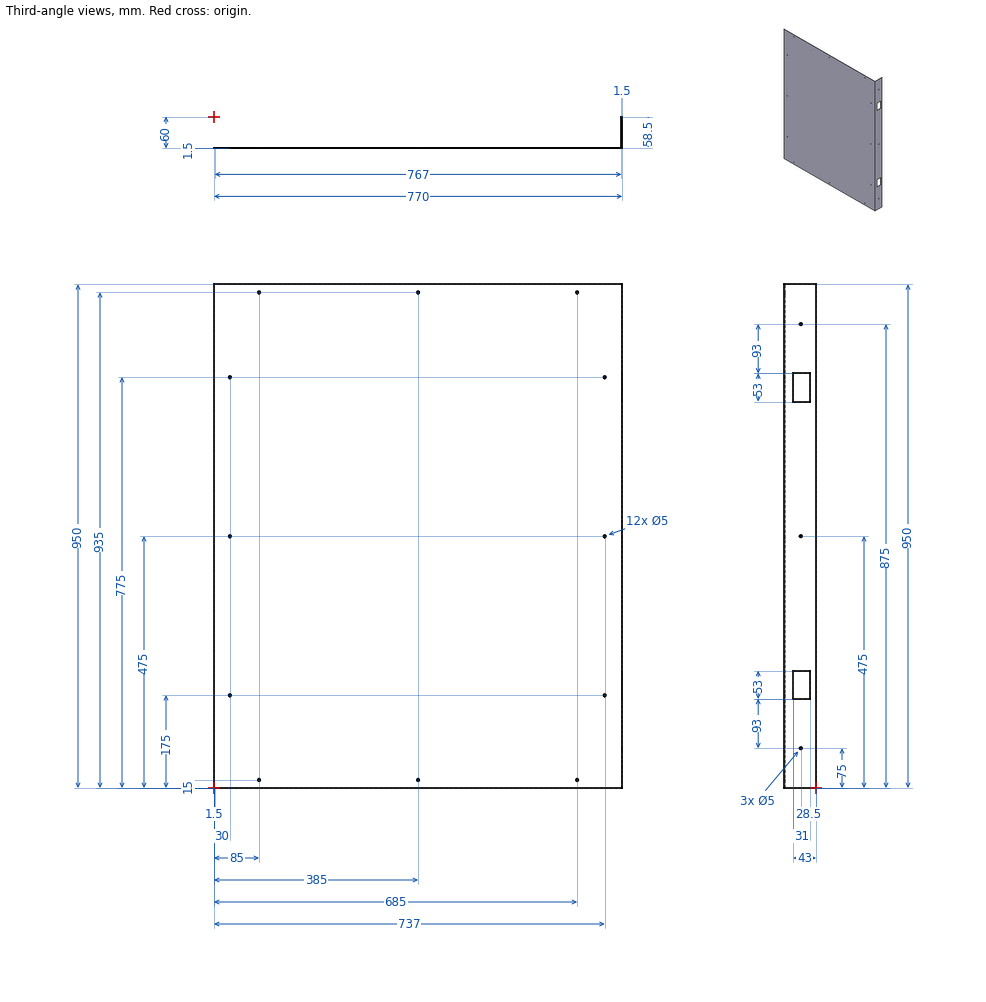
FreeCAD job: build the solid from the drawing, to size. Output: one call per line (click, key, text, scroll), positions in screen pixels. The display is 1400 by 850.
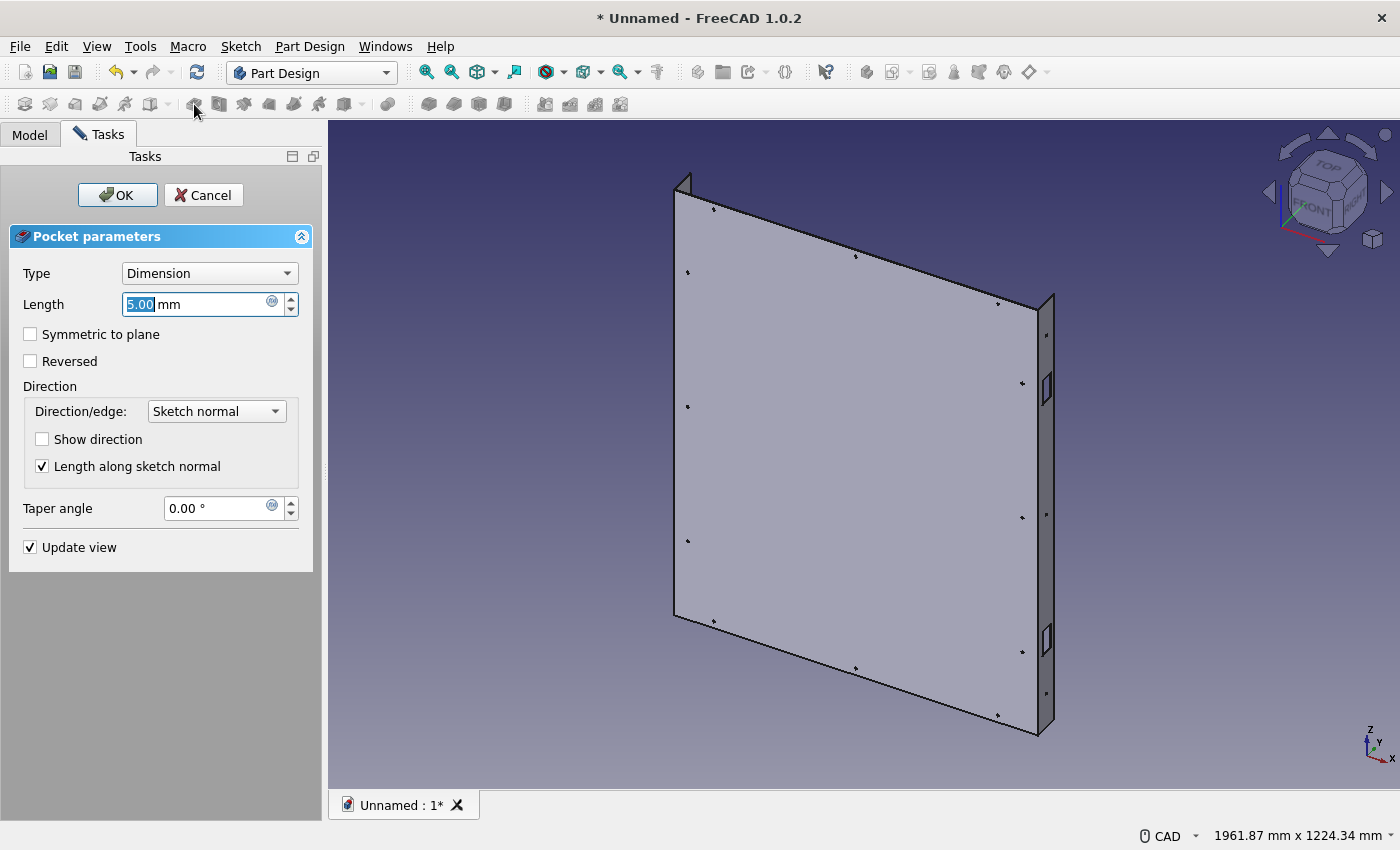
text(58.5)
key(Tab)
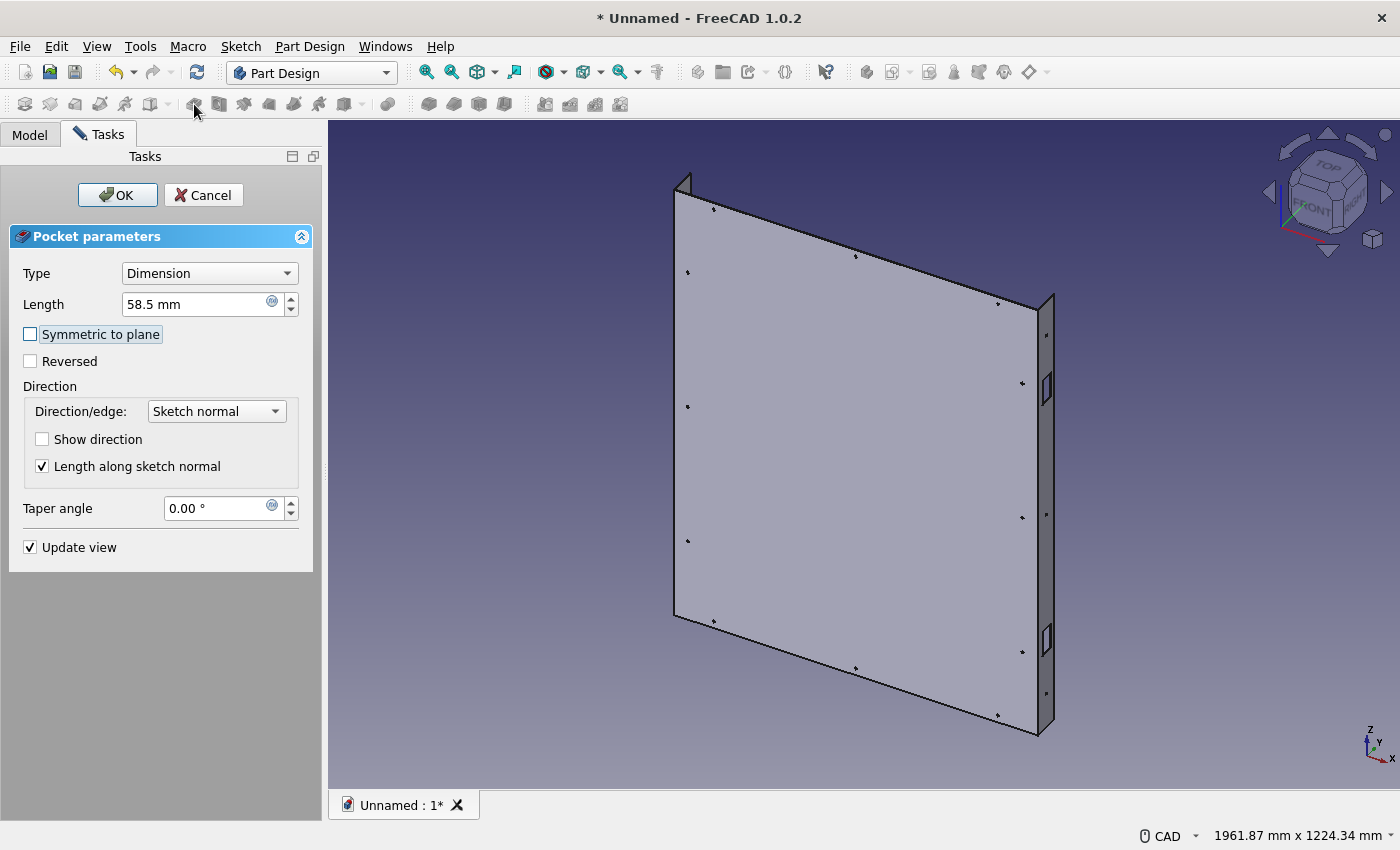
click(31, 361)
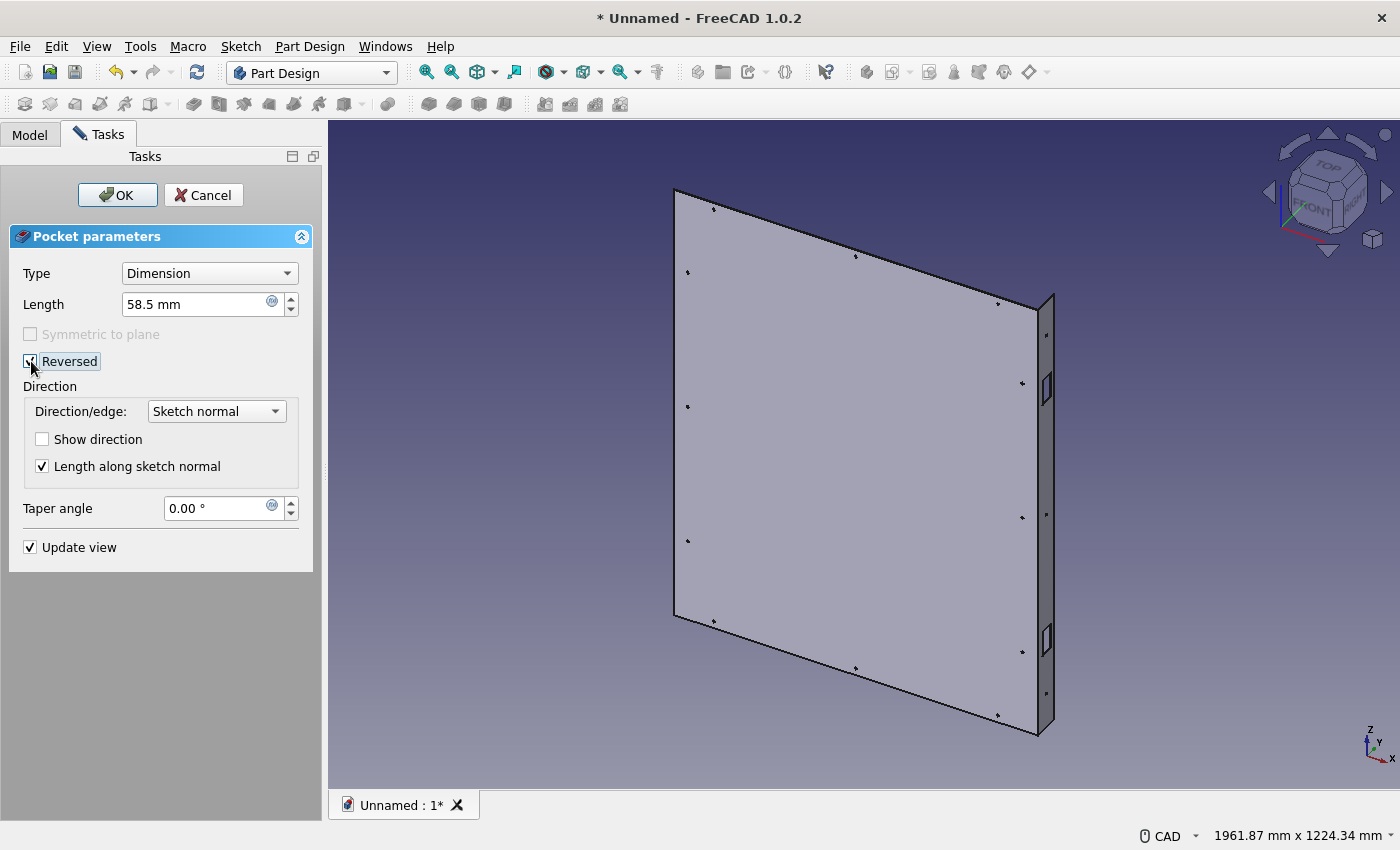
click(118, 195)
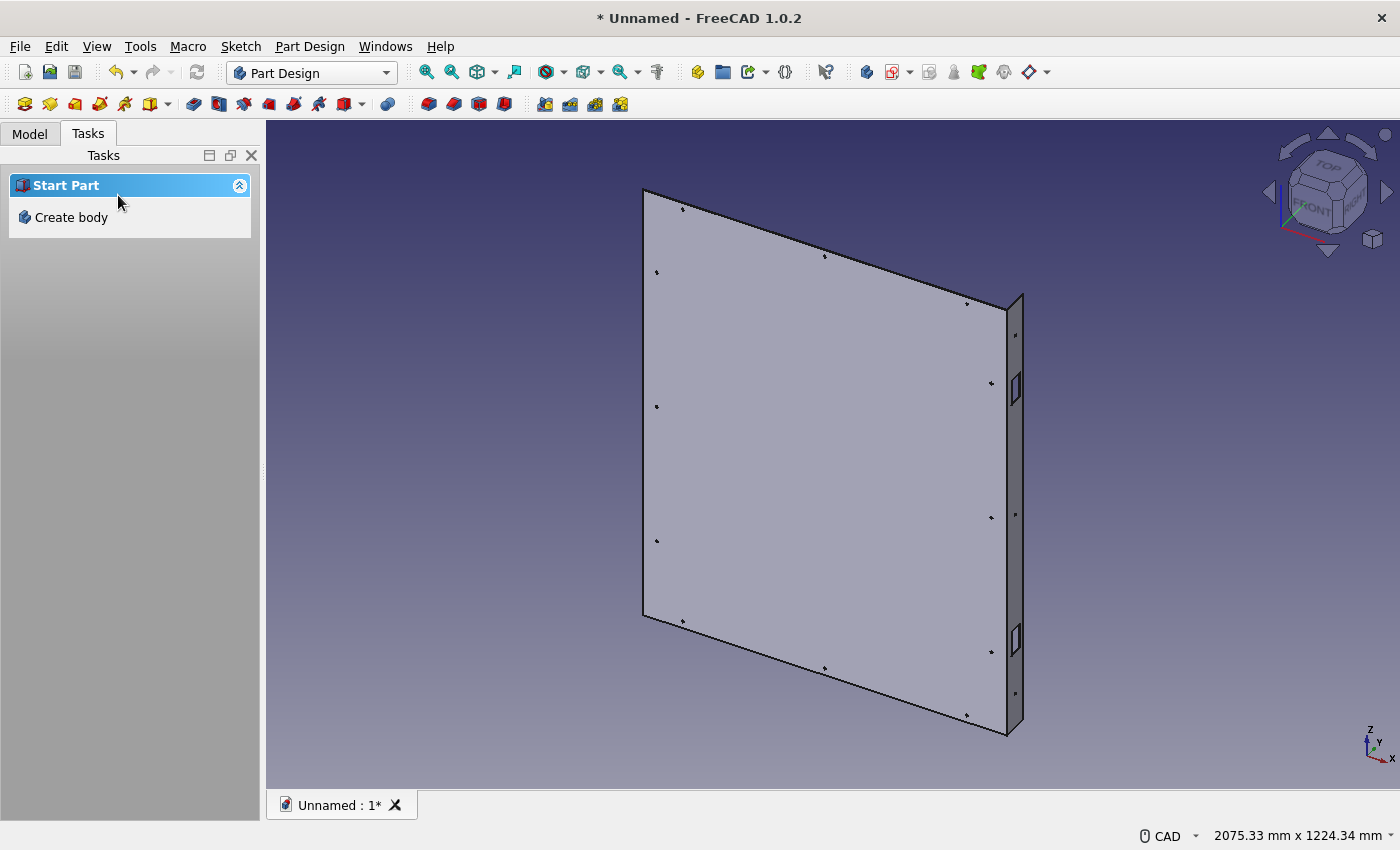
key(0)